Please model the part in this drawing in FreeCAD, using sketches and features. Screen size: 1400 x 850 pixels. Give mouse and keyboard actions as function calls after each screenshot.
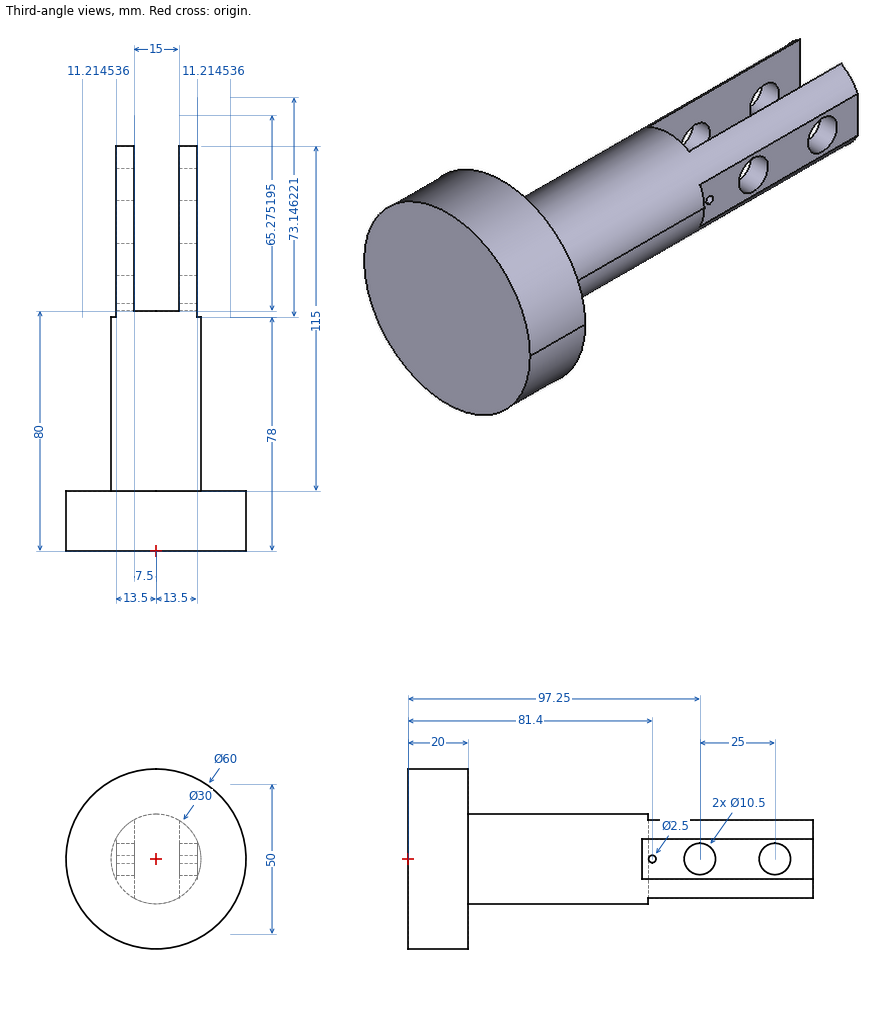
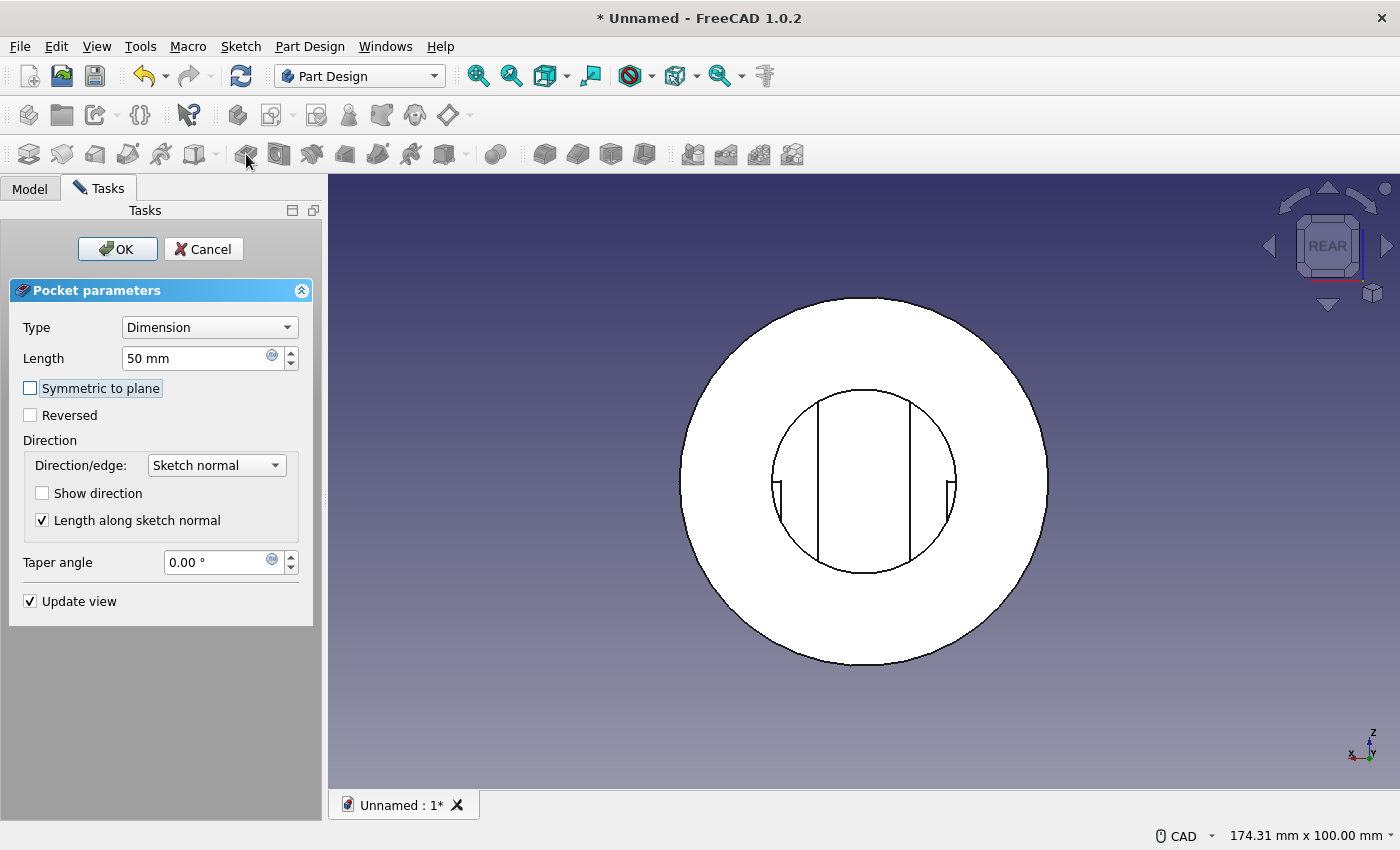
click(31, 388)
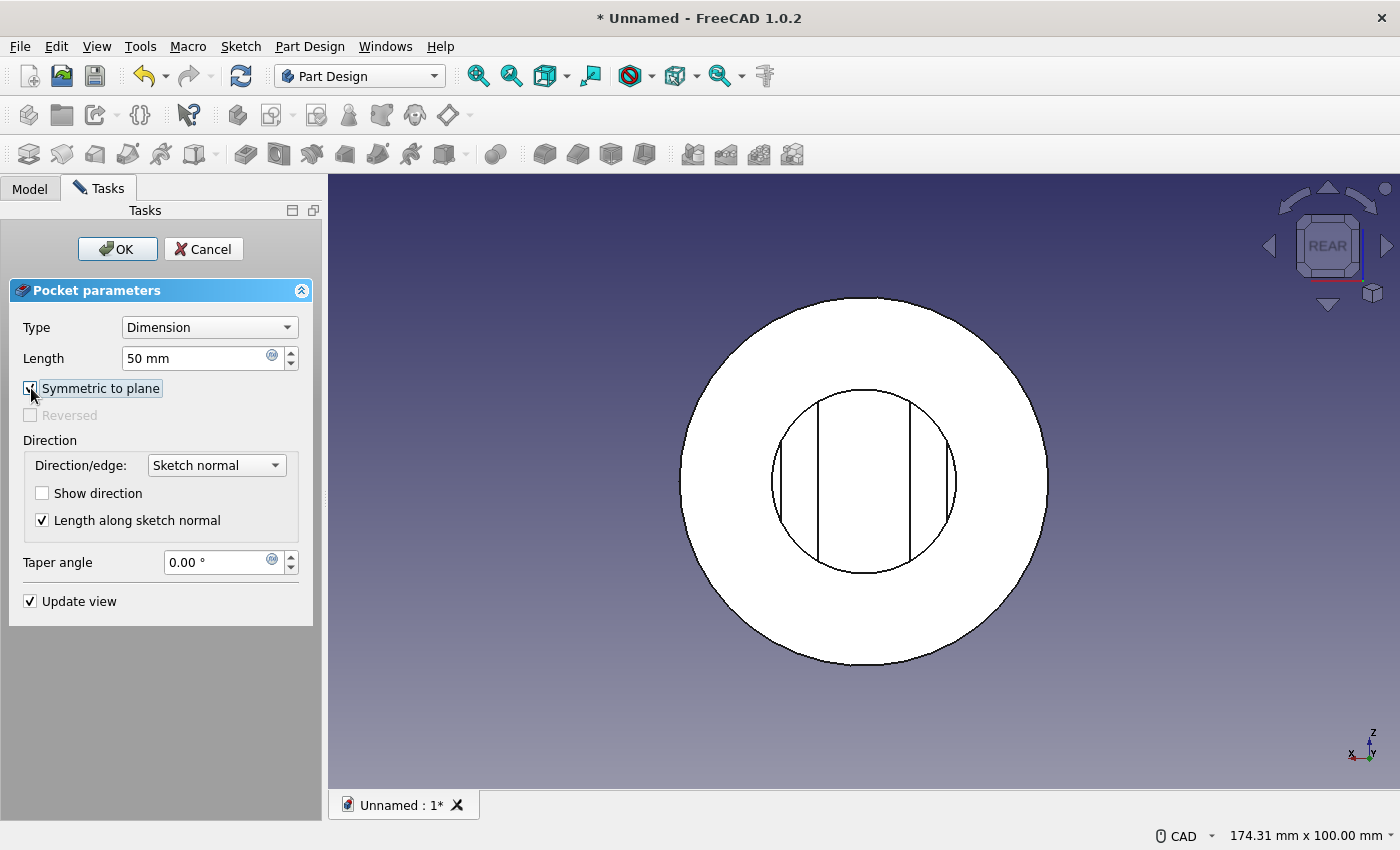
click(118, 249)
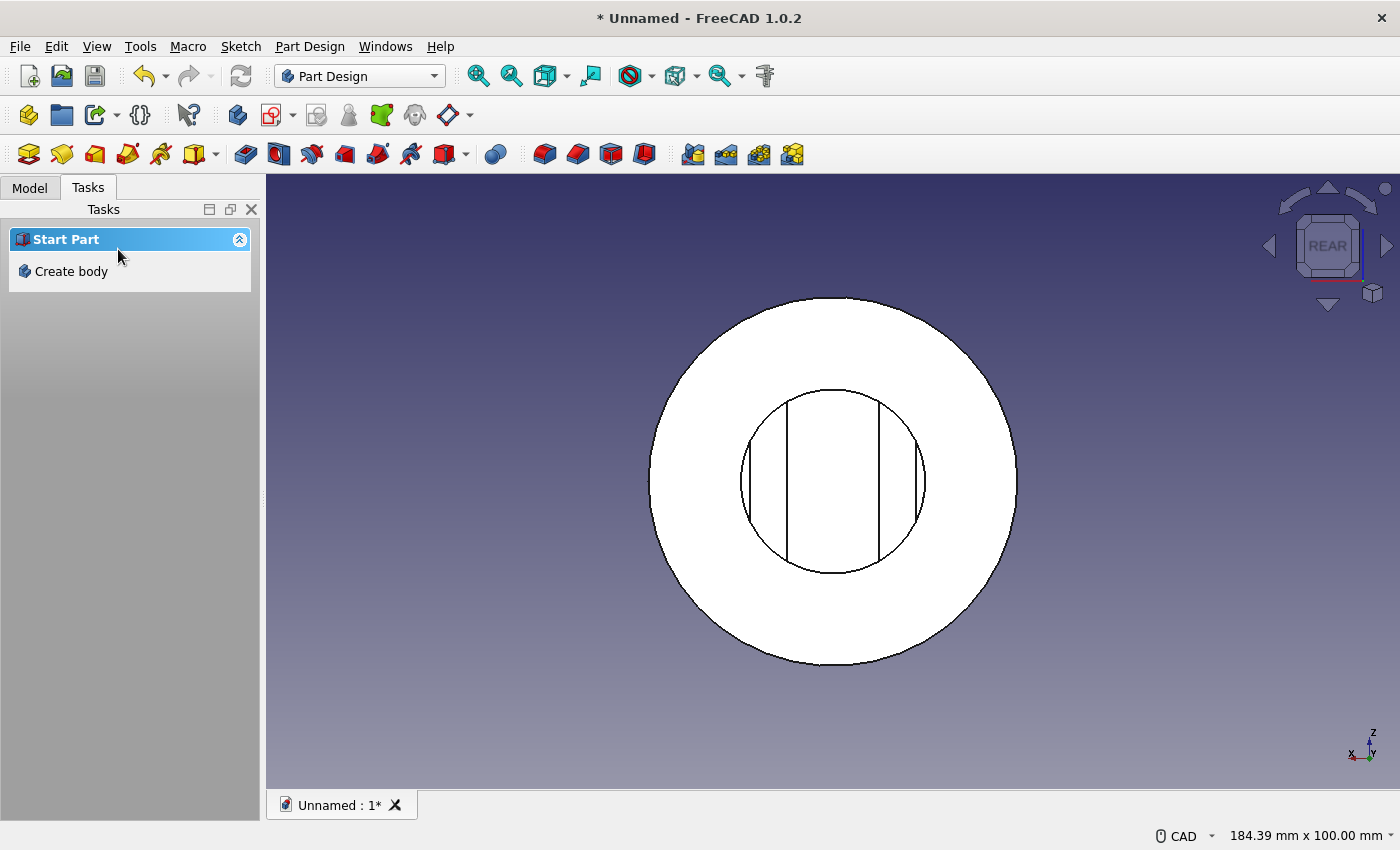
key(0)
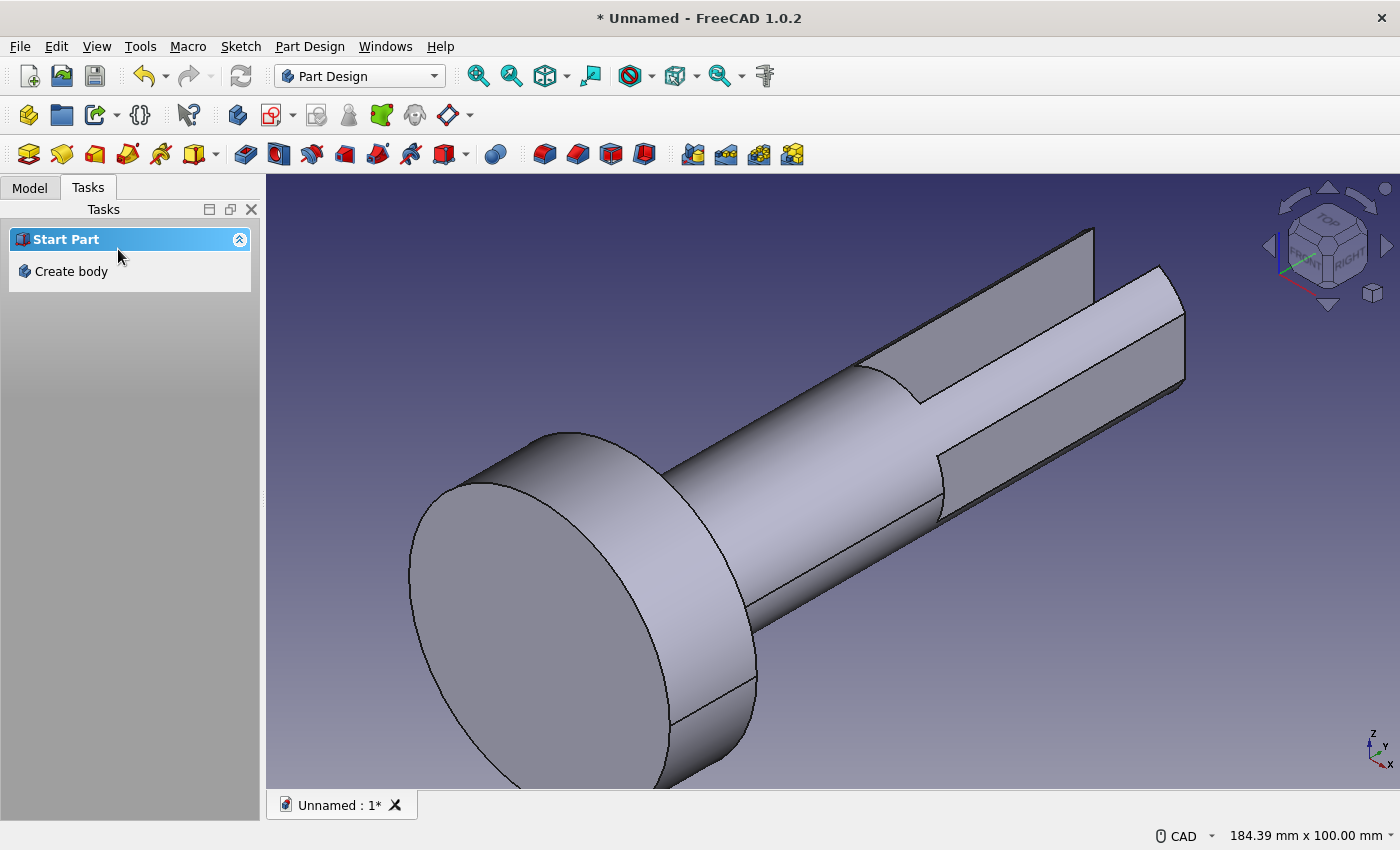
click(479, 76)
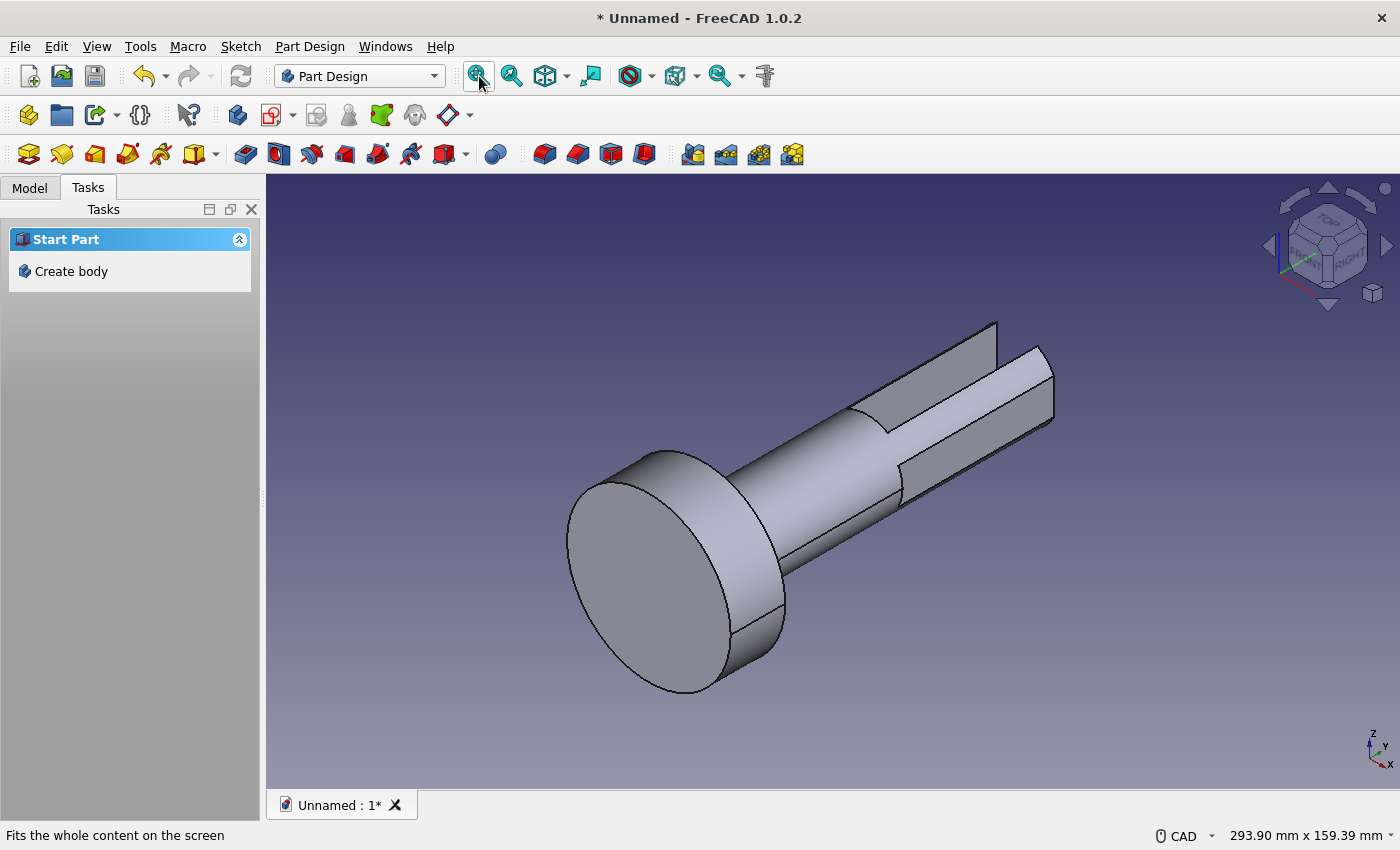
click(1021, 415)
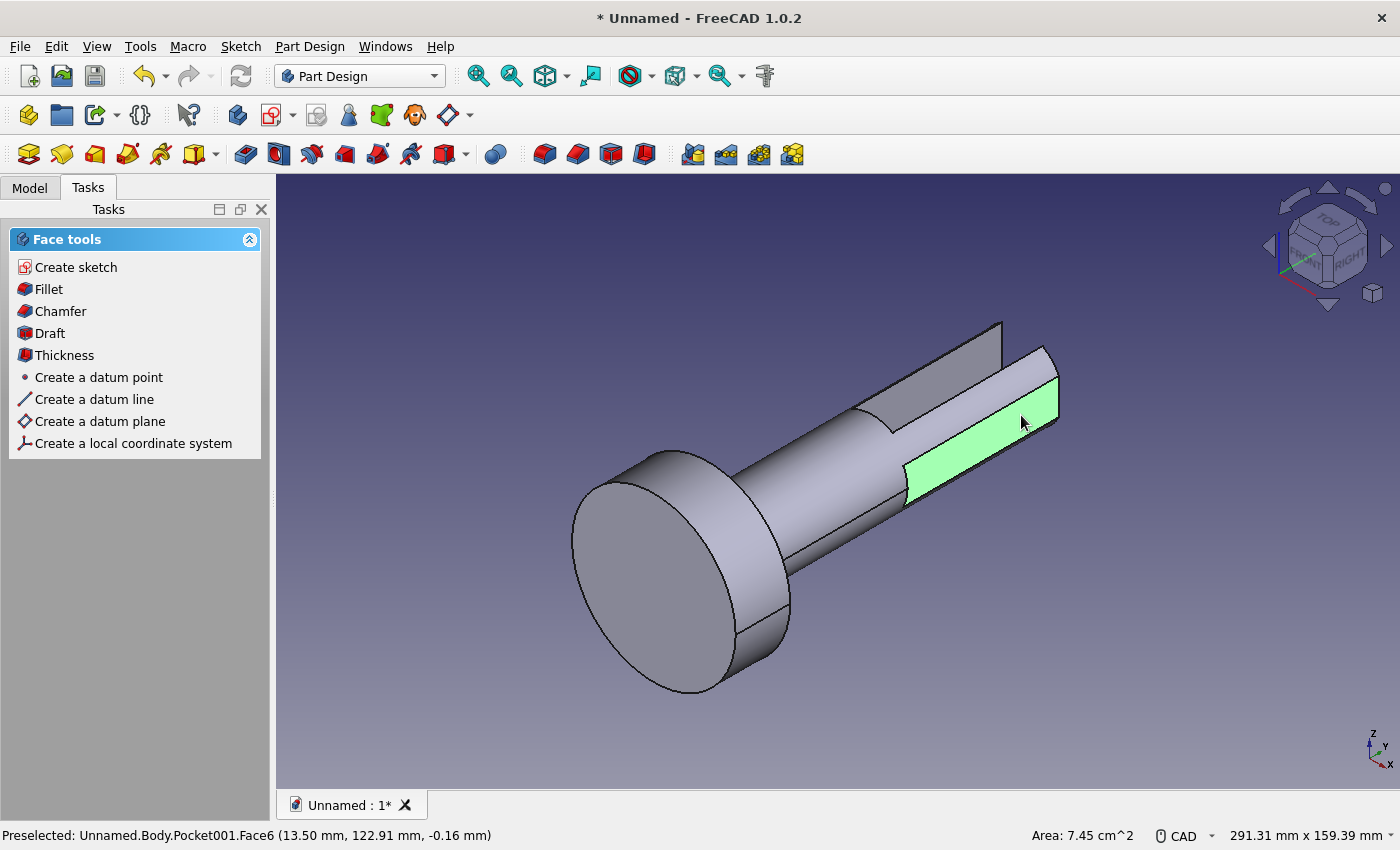
click(270, 116)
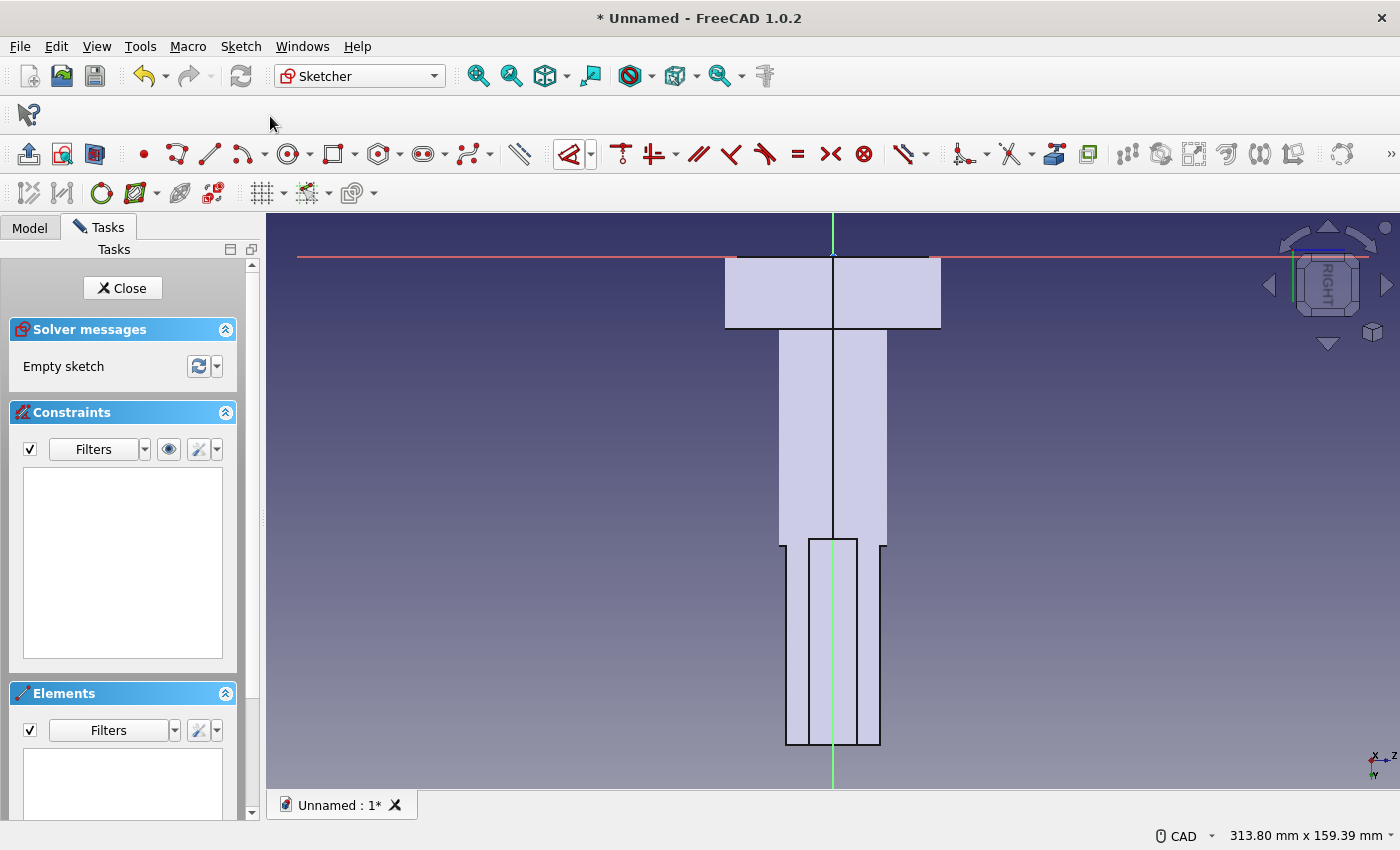
key(q)
key(s)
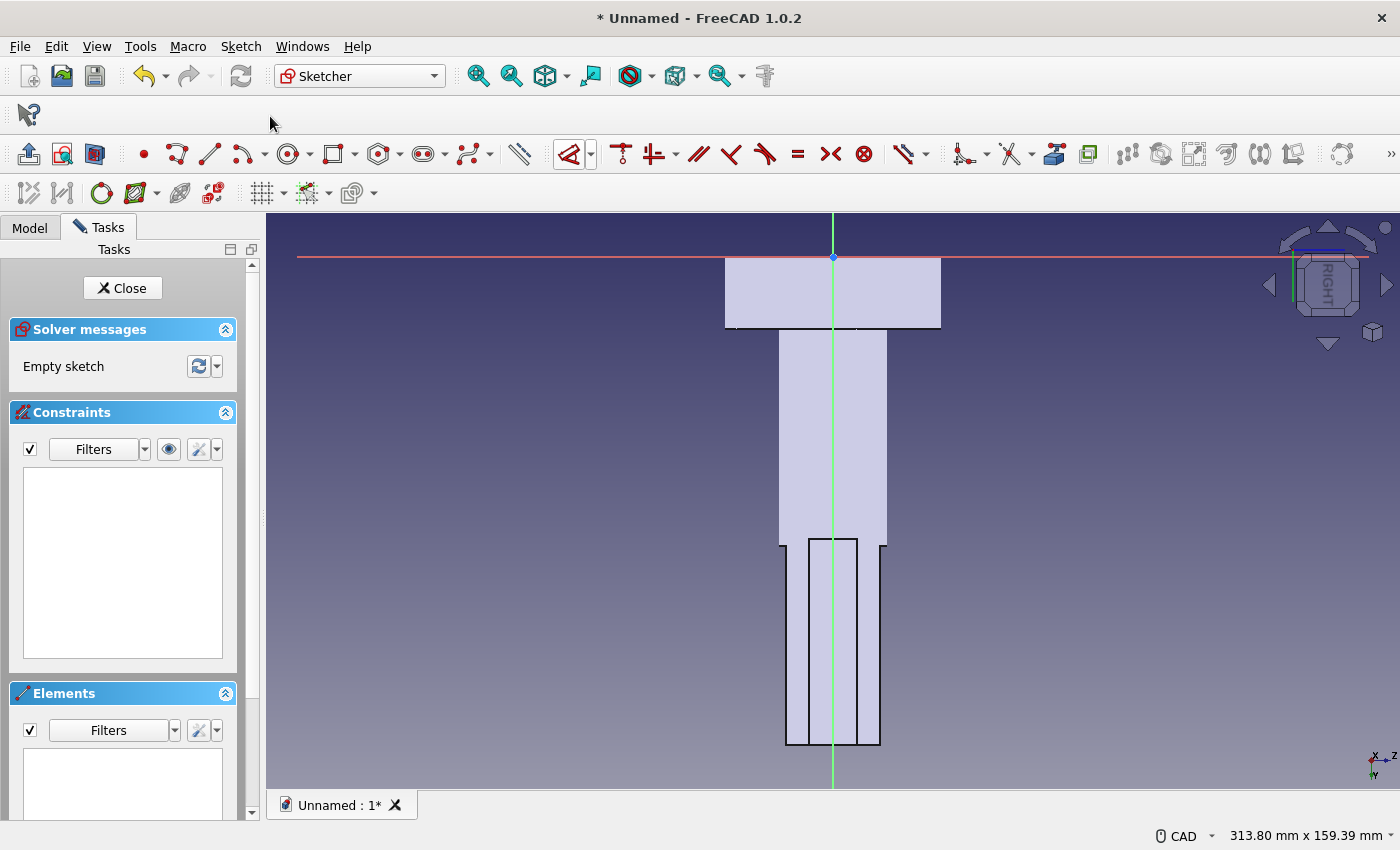
scroll(873, 743, up, 5)